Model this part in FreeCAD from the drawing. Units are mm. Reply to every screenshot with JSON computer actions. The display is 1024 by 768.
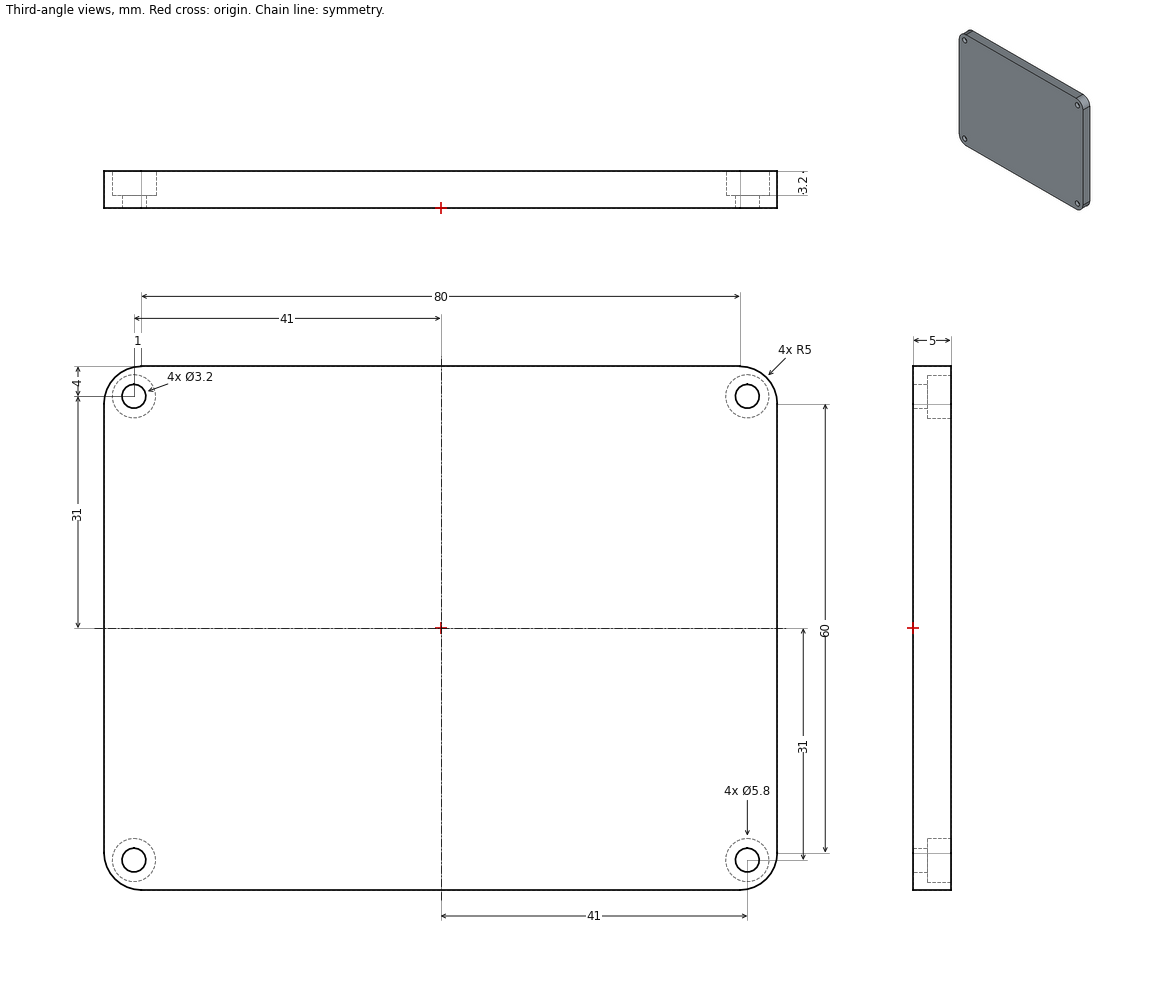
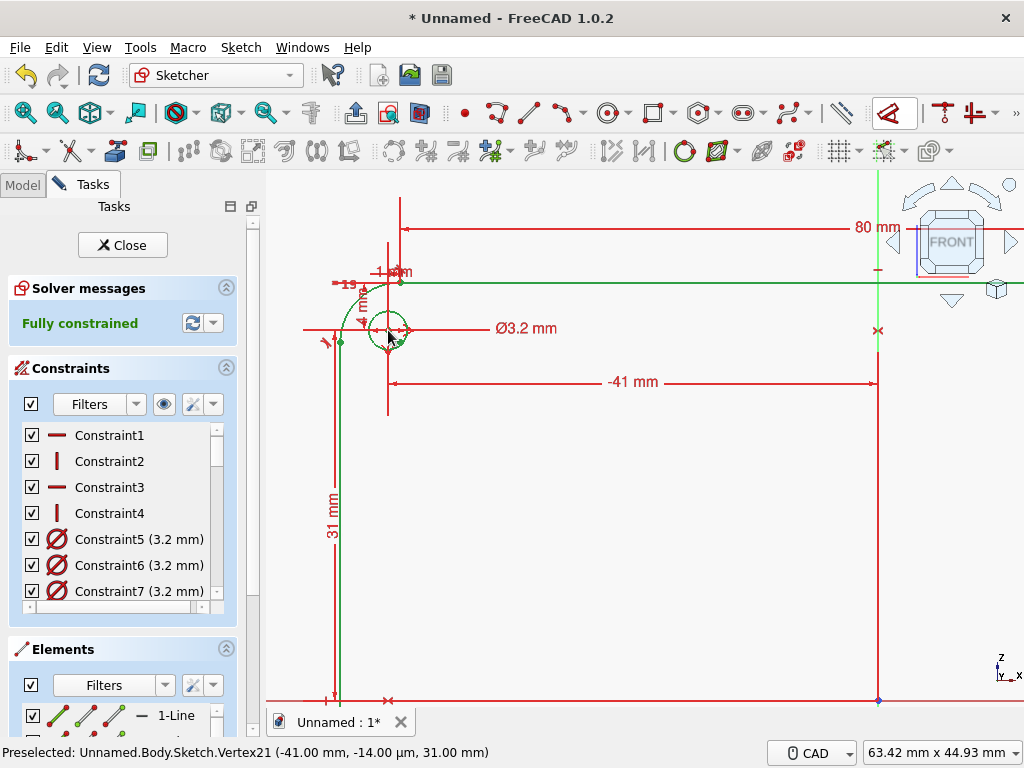
{"action": "left_click", "coordinate": [123, 245]}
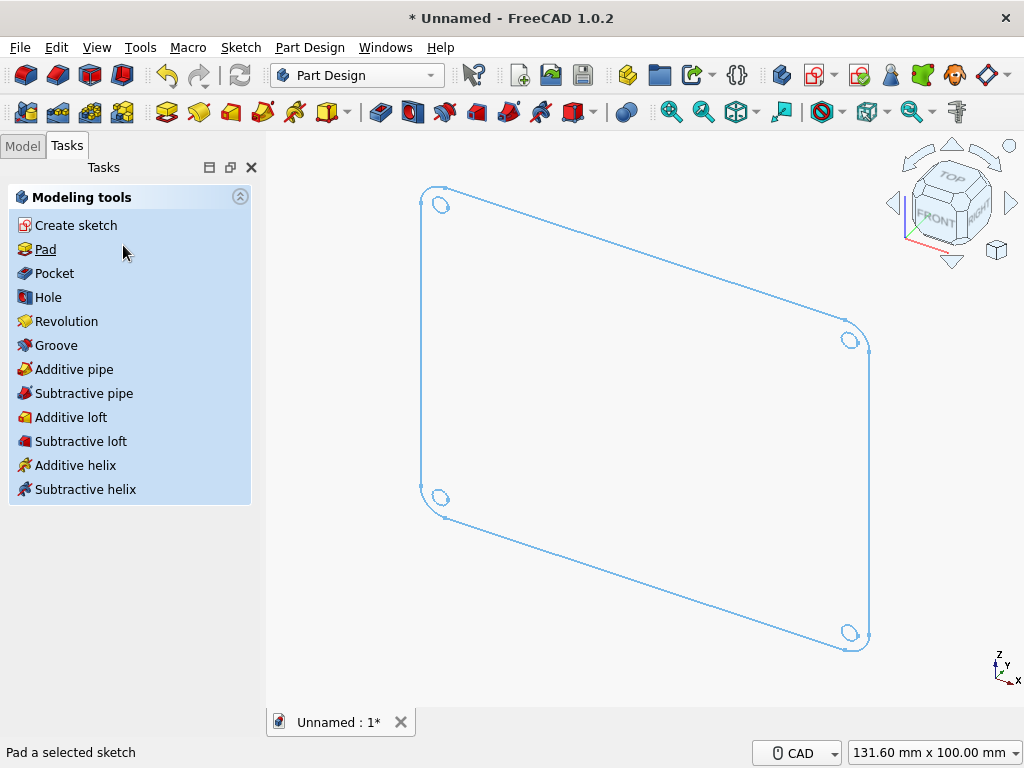
{"action": "left_click", "coordinate": [168, 112]}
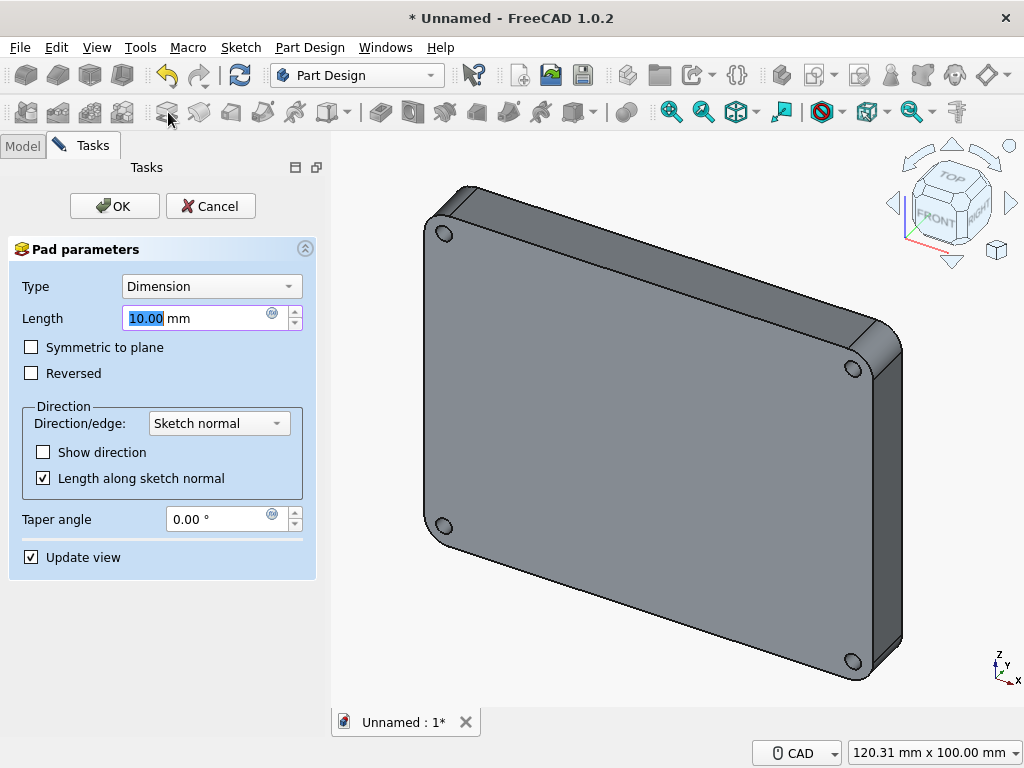
{"action": "type", "text": "5"}
{"action": "key", "text": "Tab"}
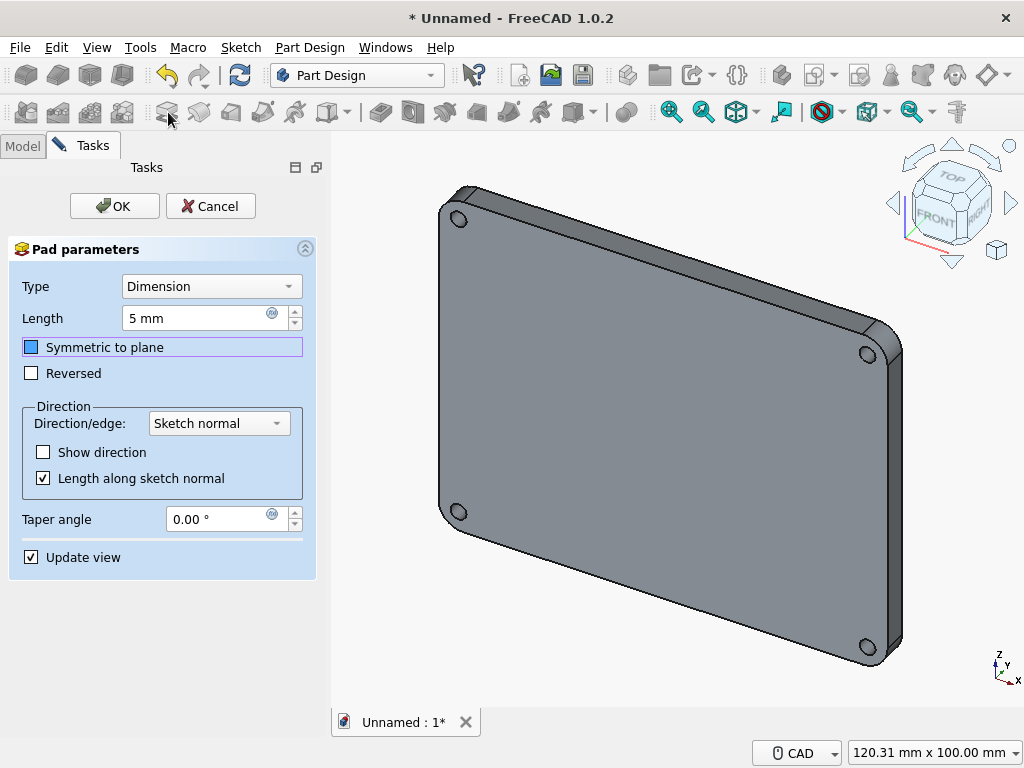
{"action": "left_click", "coordinate": [30, 373]}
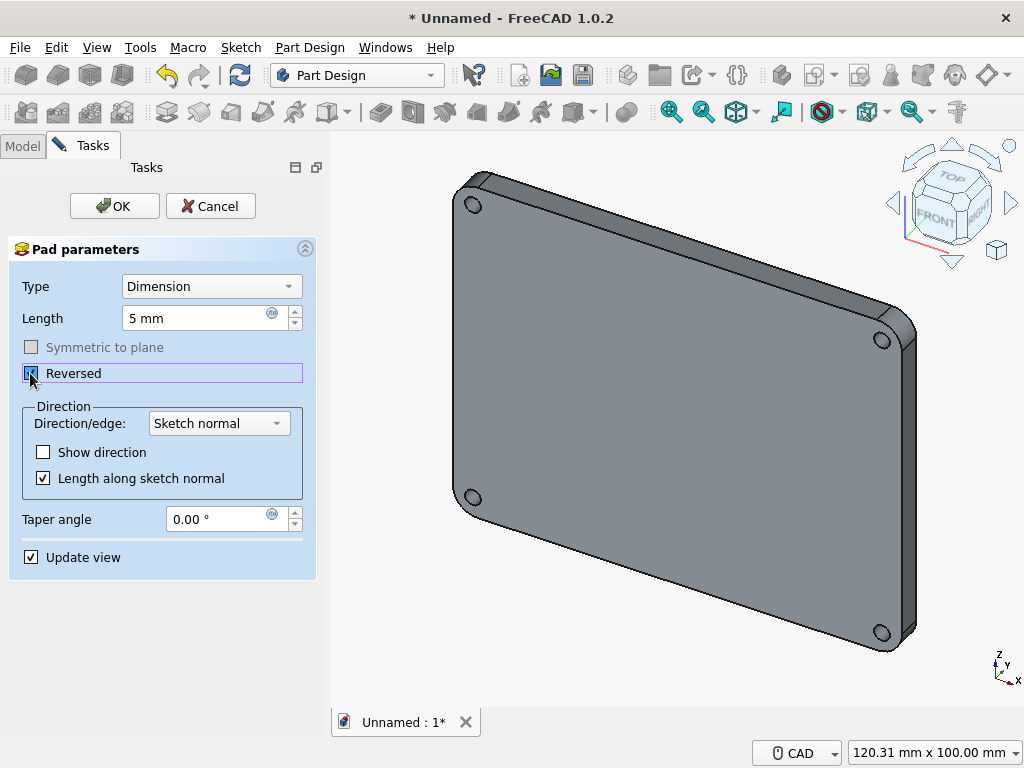
{"action": "left_click", "coordinate": [115, 206]}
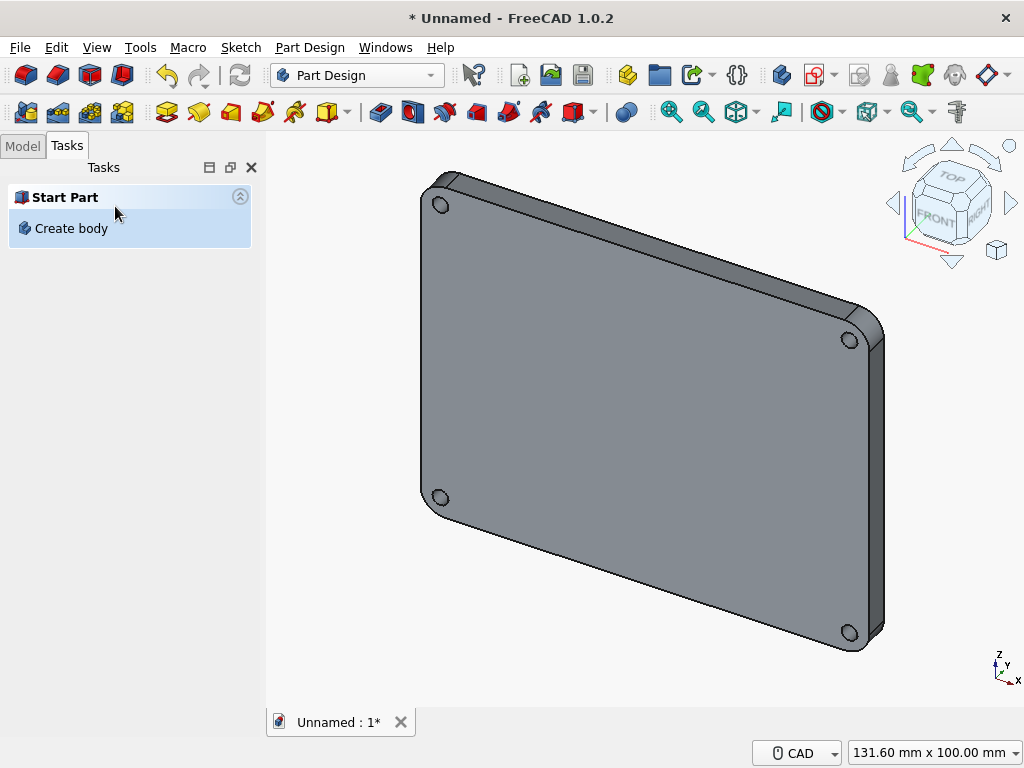
{"action": "key", "text": "4"}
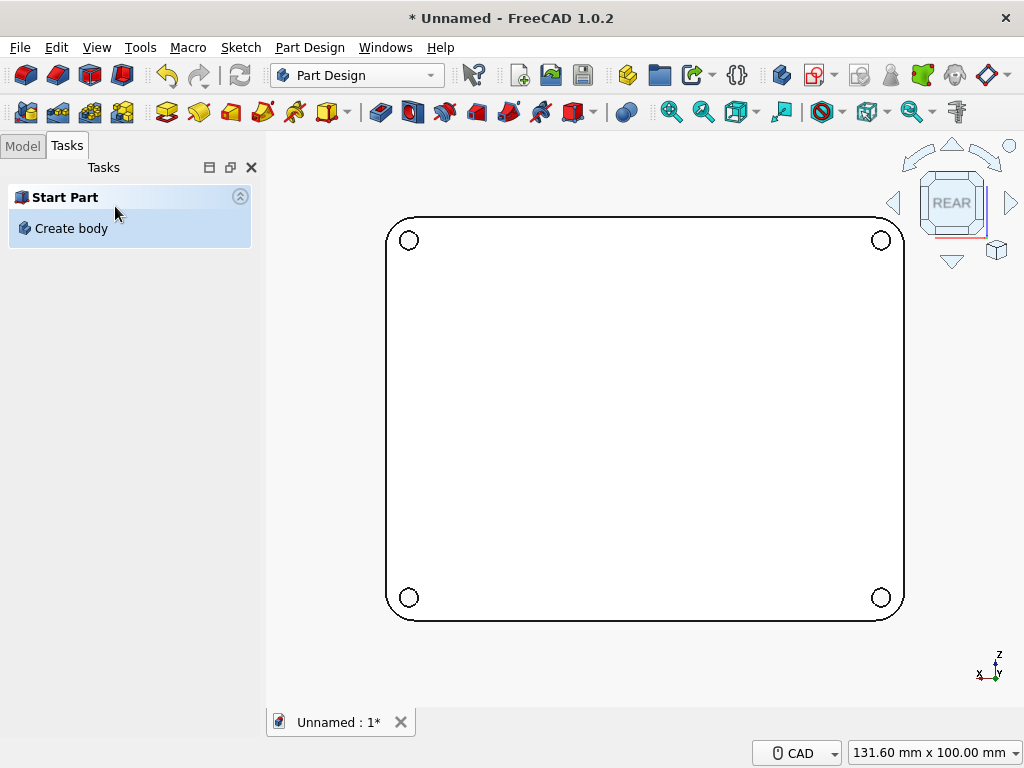
{"action": "left_click", "coordinate": [645, 418]}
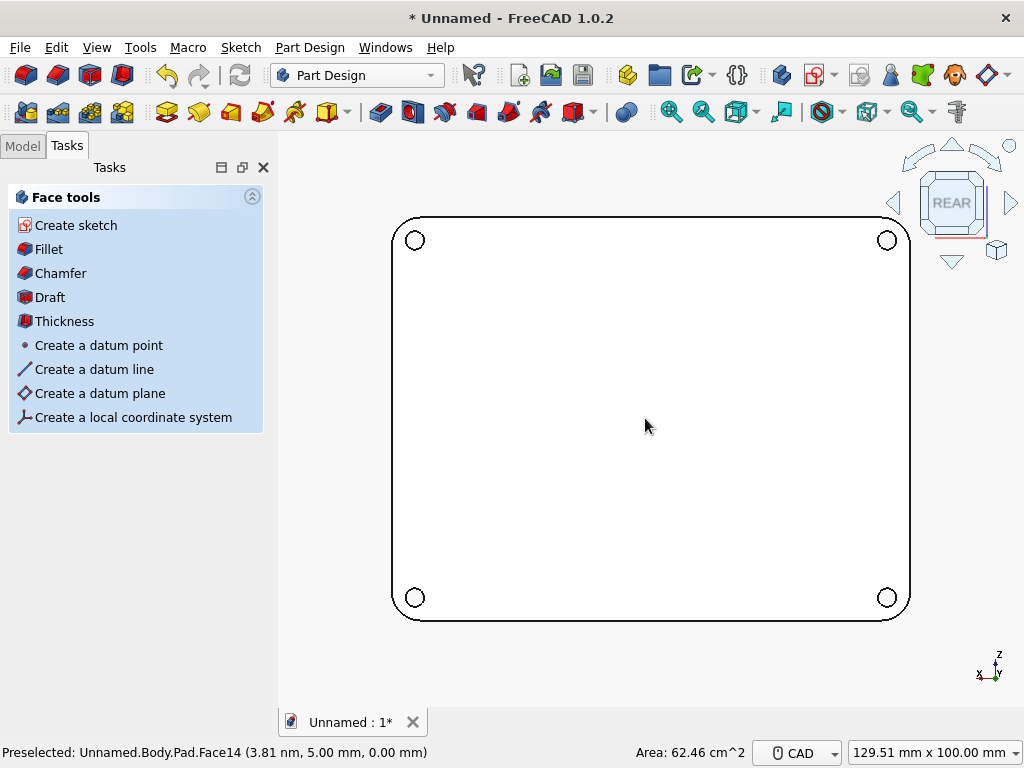
{"action": "left_click", "coordinate": [814, 76]}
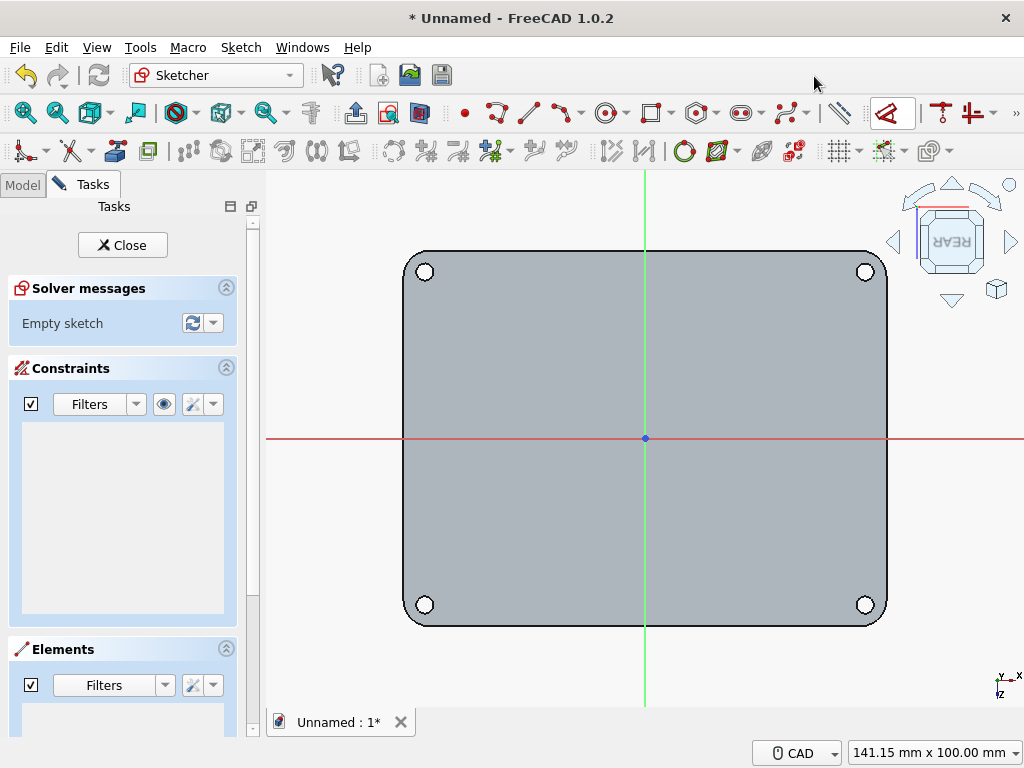
{"action": "scroll", "coordinate": [294, 438], "scroll_direction": "down", "scroll_amount": 1}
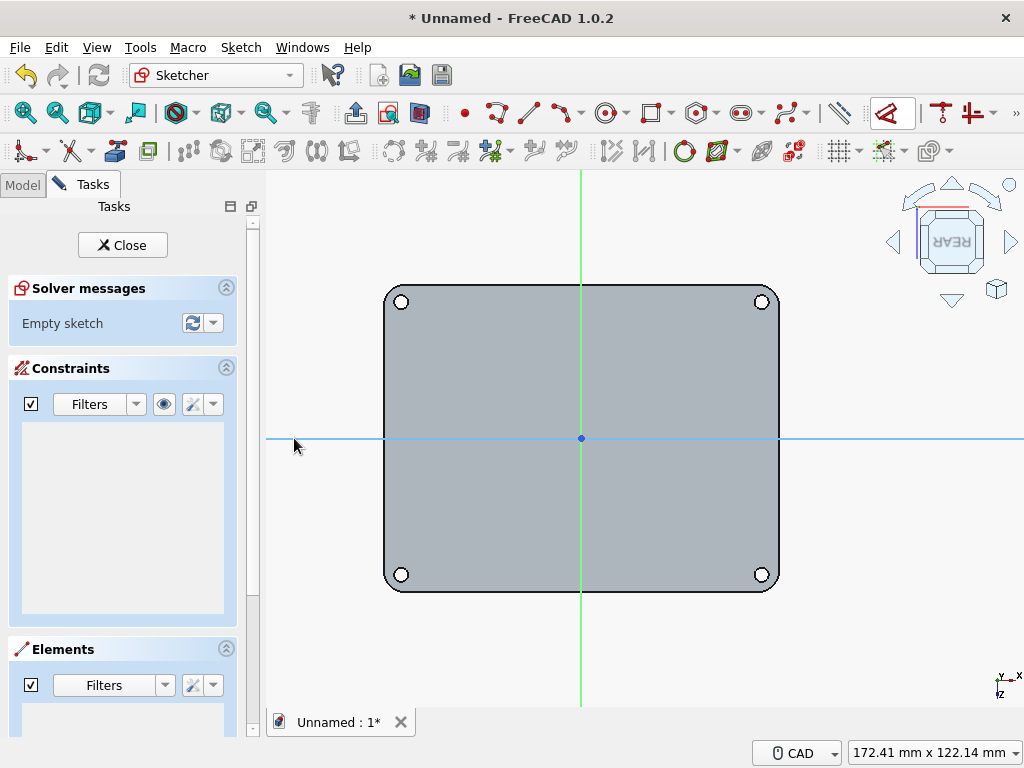
{"action": "key", "text": "g c"}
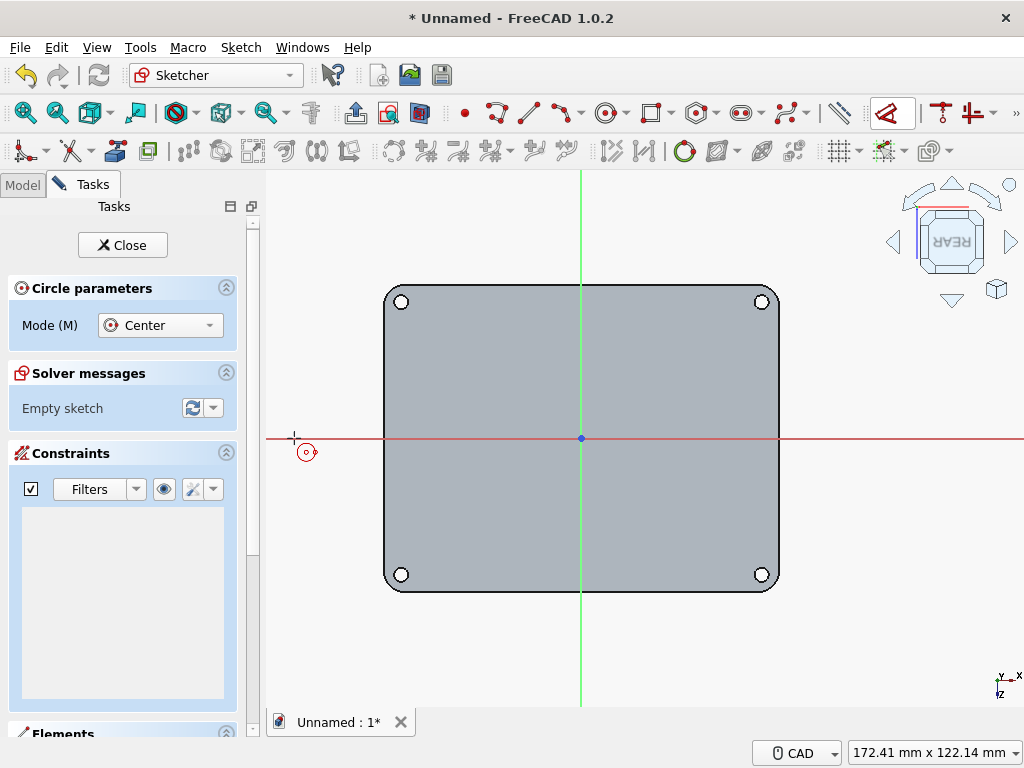
{"action": "scroll", "coordinate": [762, 302], "scroll_direction": "up", "scroll_amount": 3}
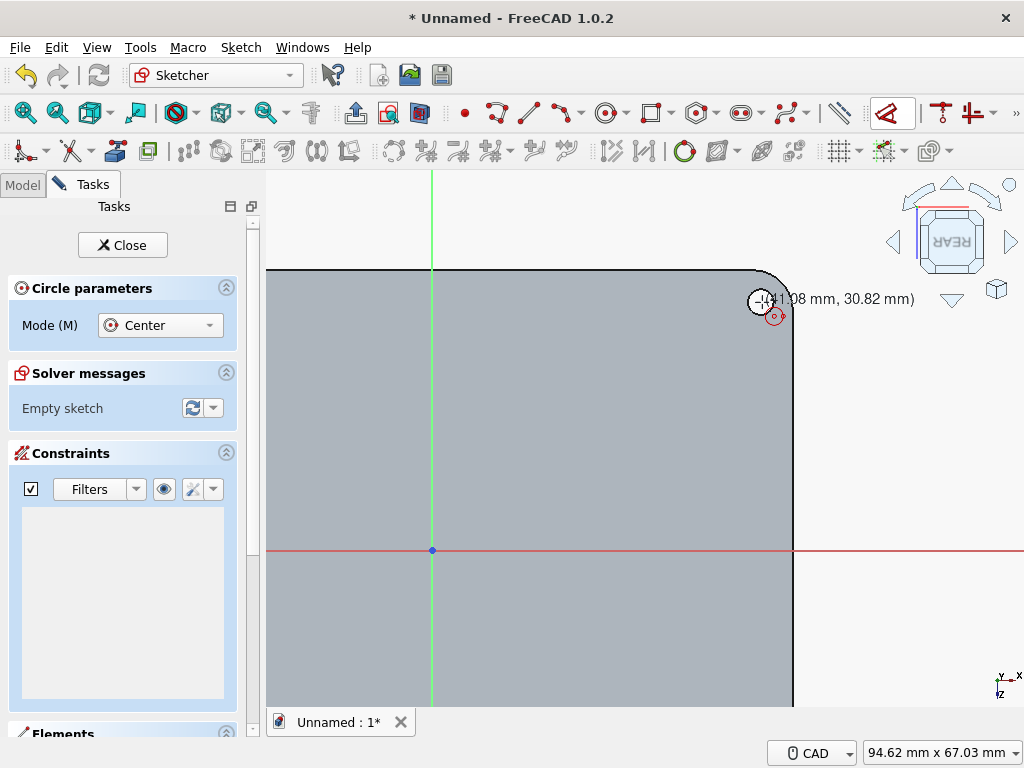
{"action": "left_click", "coordinate": [761, 302]}
{"action": "mouse_move", "coordinate": [777, 286]}